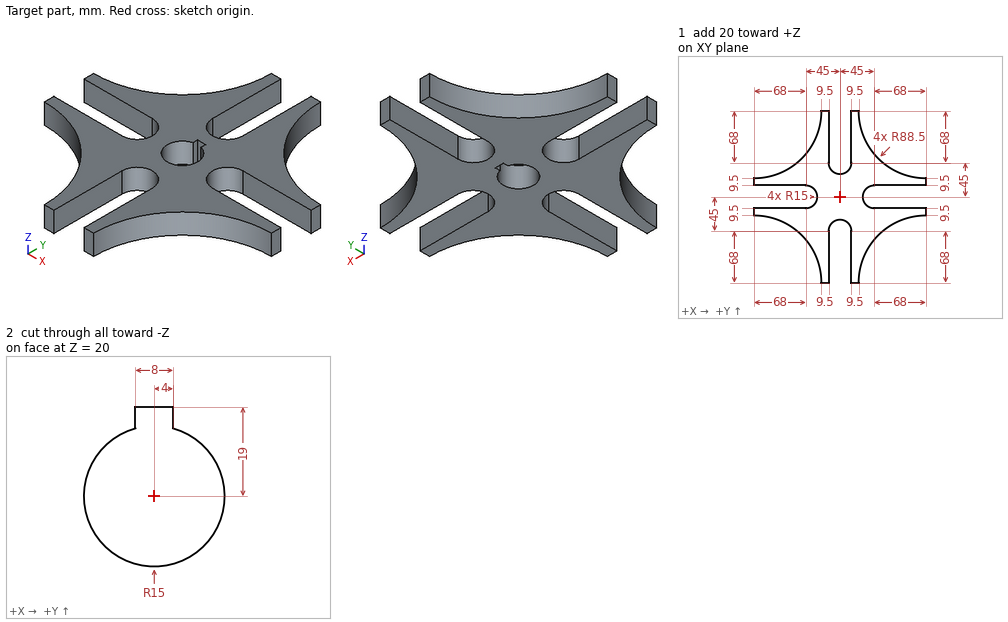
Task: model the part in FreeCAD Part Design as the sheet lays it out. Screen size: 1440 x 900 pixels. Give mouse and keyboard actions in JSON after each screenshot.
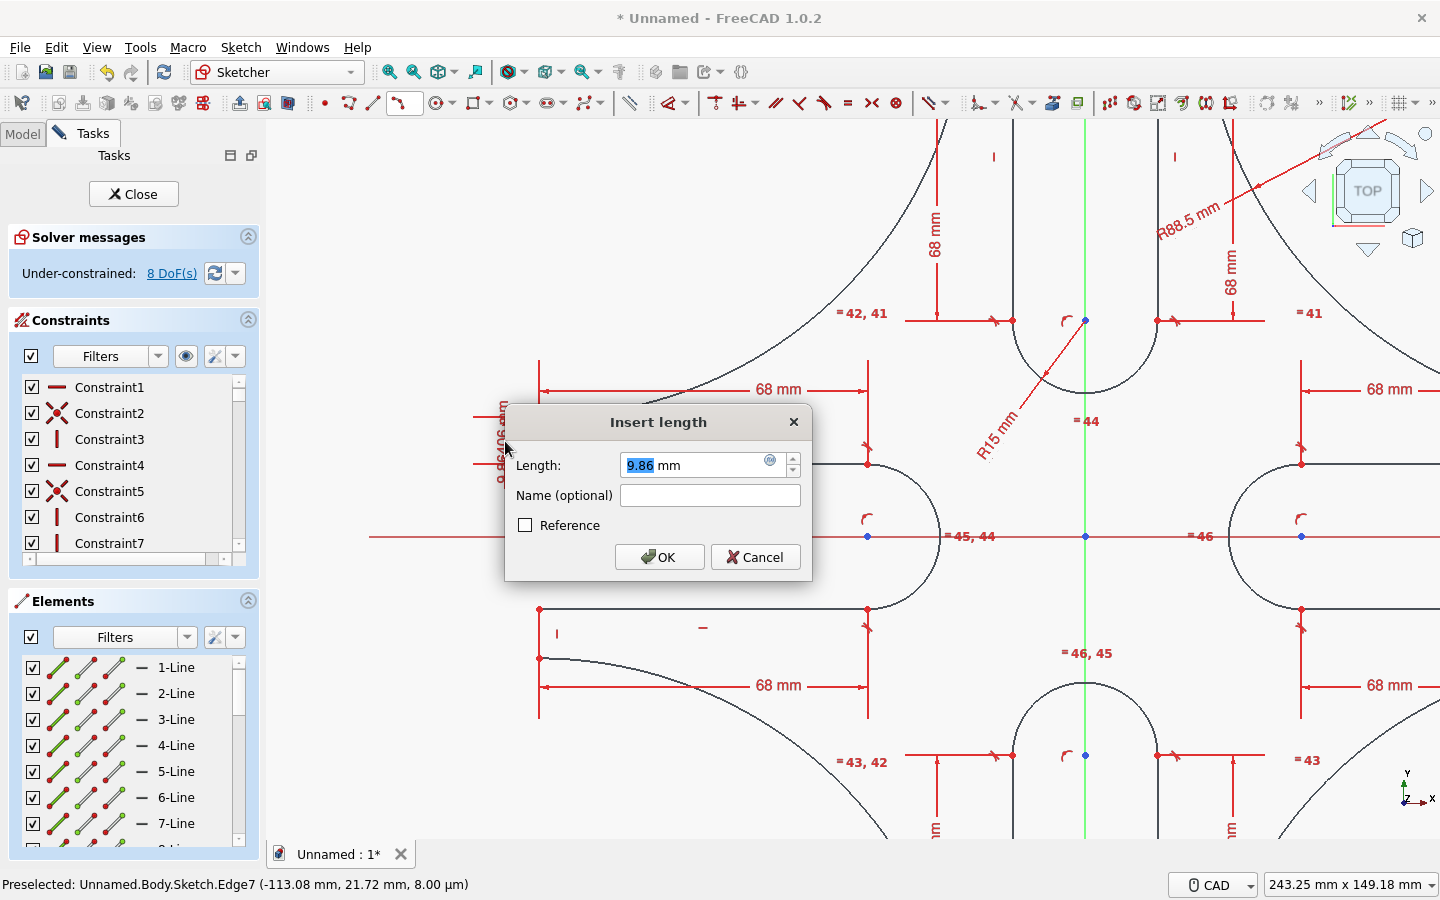
{"action": "type", "text": "9.5"}
{"action": "key", "text": "Return"}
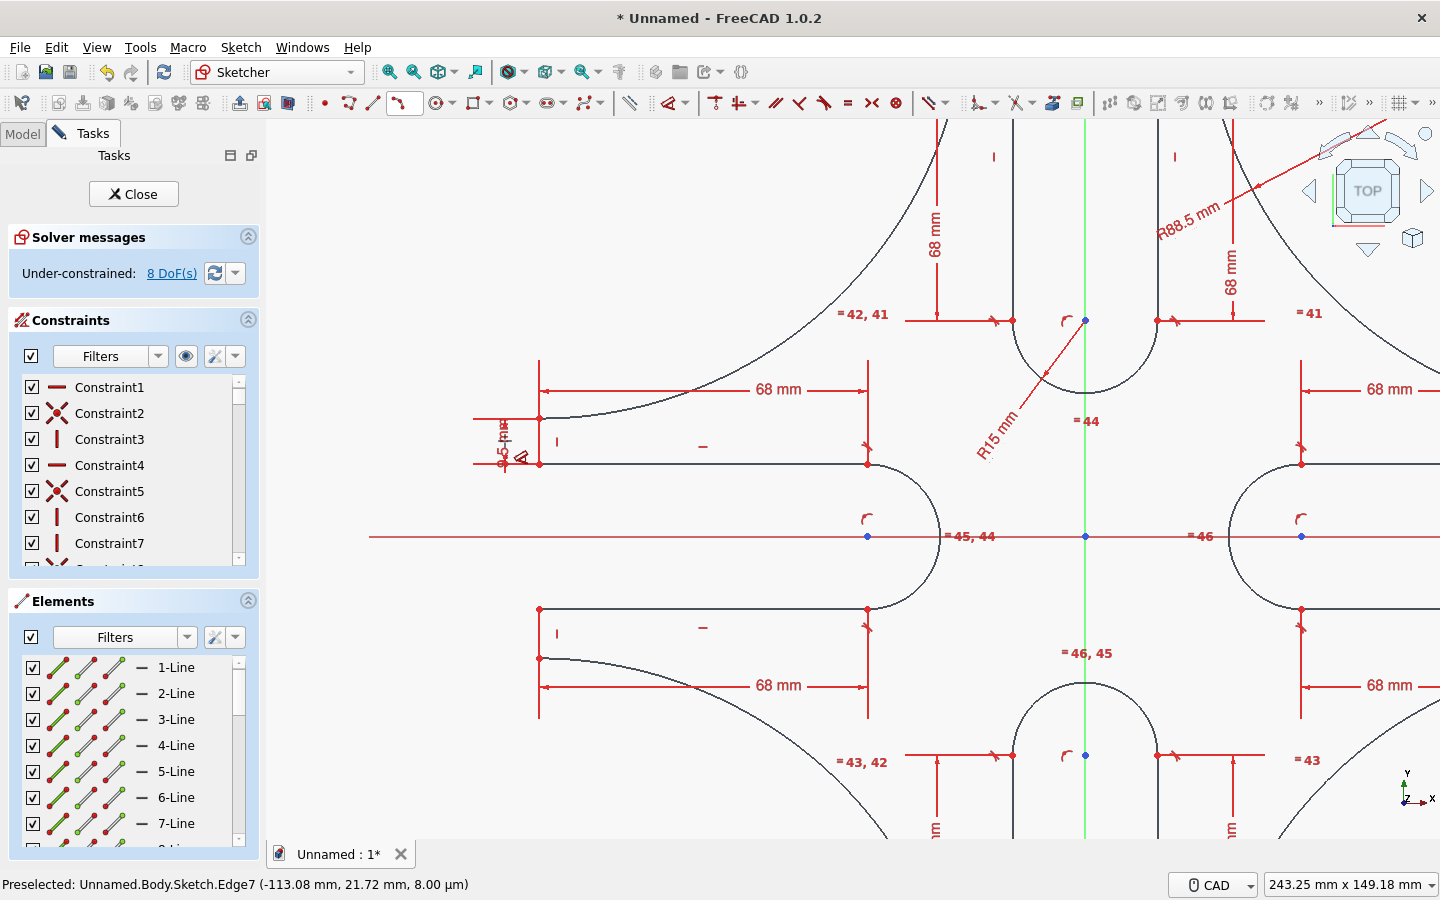
{"action": "left_click", "coordinate": [539, 624]}
{"action": "left_click", "coordinate": [505, 634]}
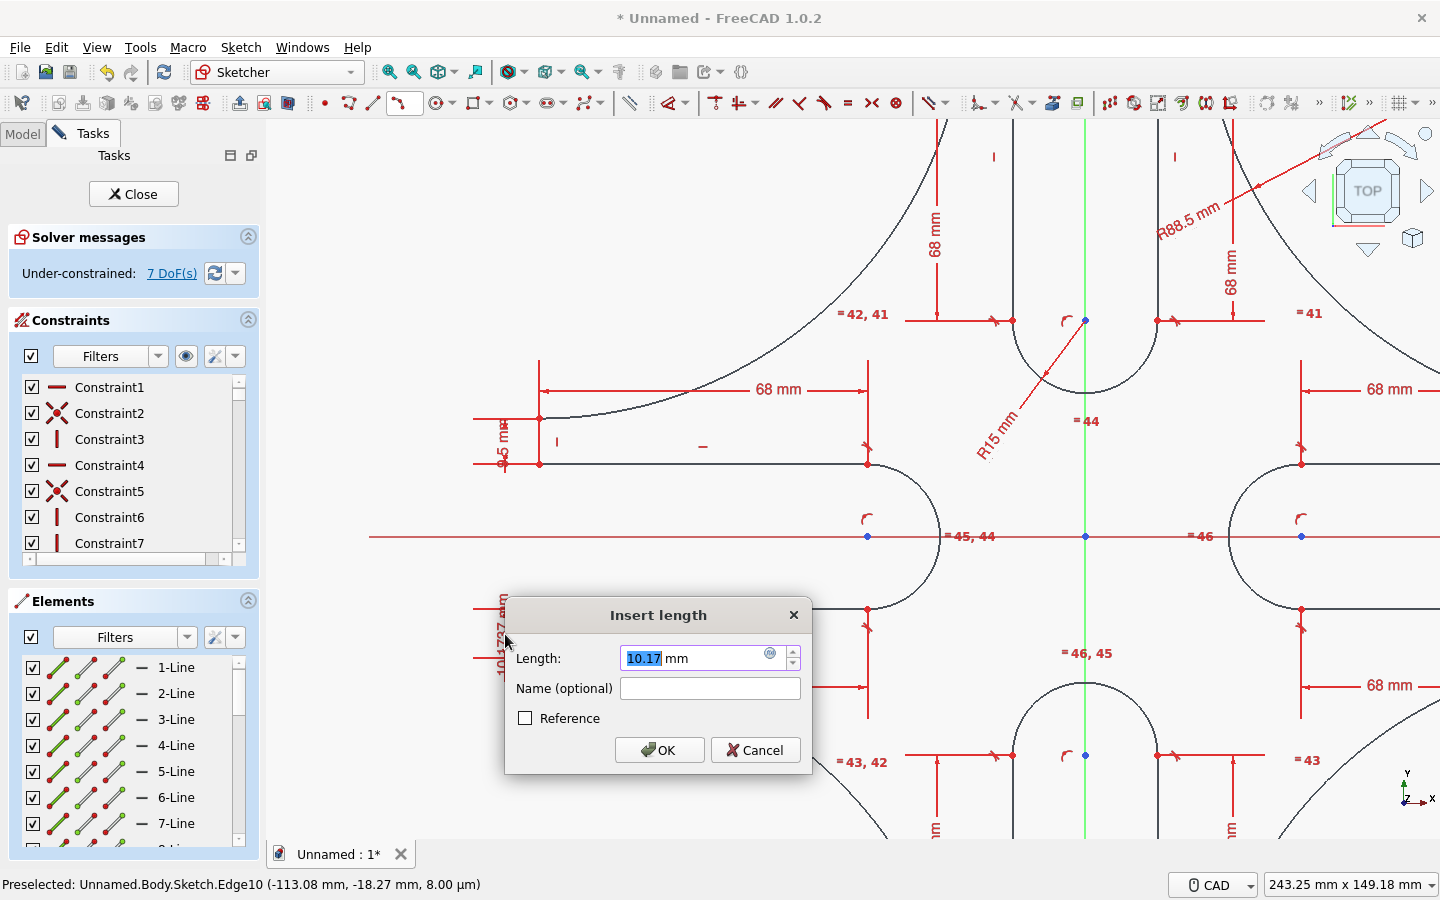
{"action": "type", "text": "9.5"}
{"action": "key", "text": "Return"}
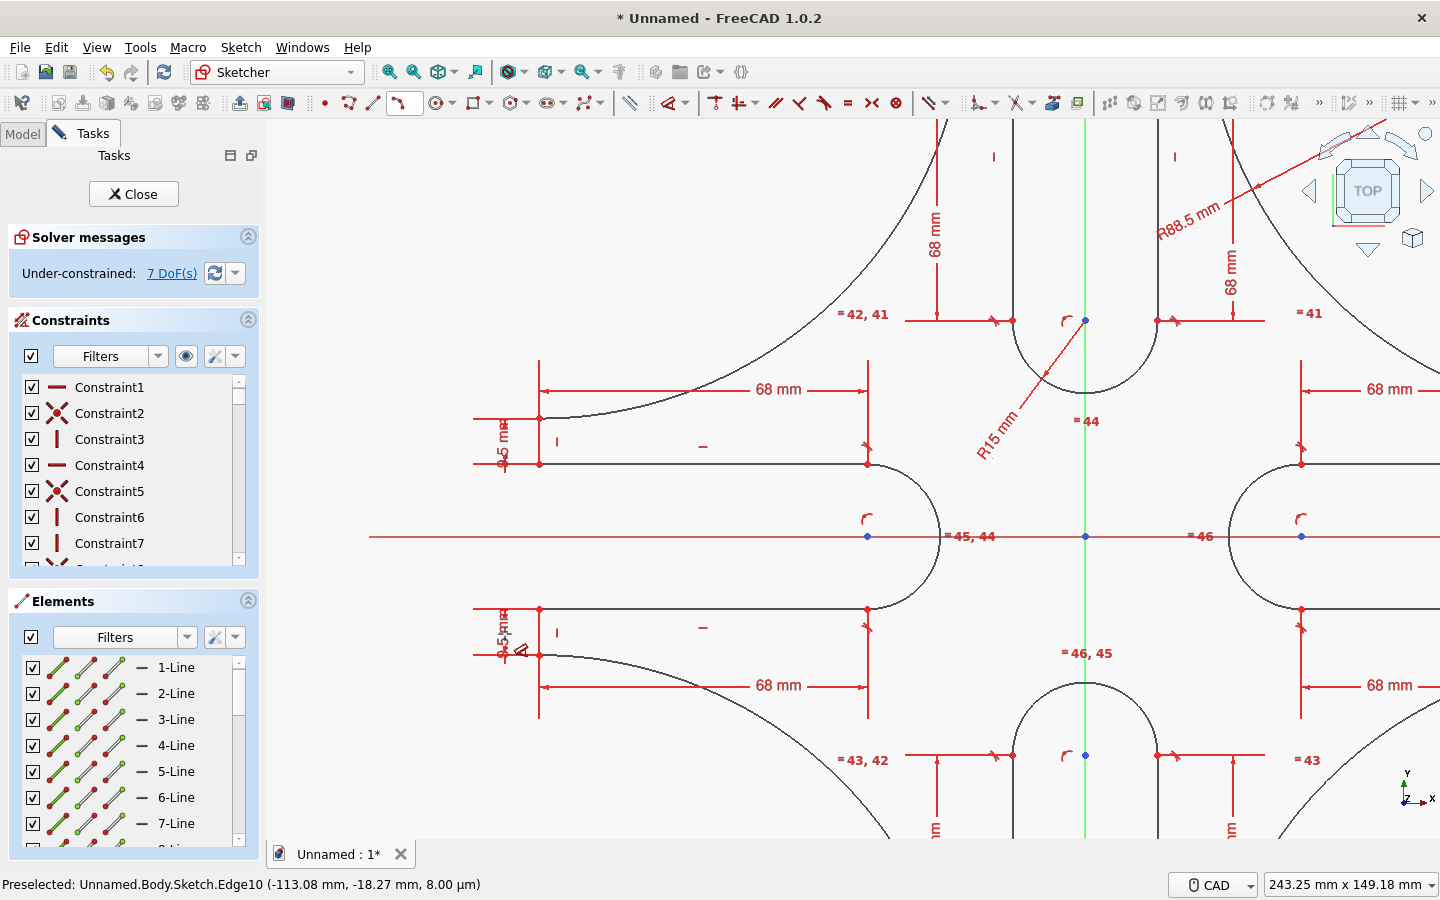
{"action": "scroll", "coordinate": [539, 432], "scroll_direction": "down", "scroll_amount": 4}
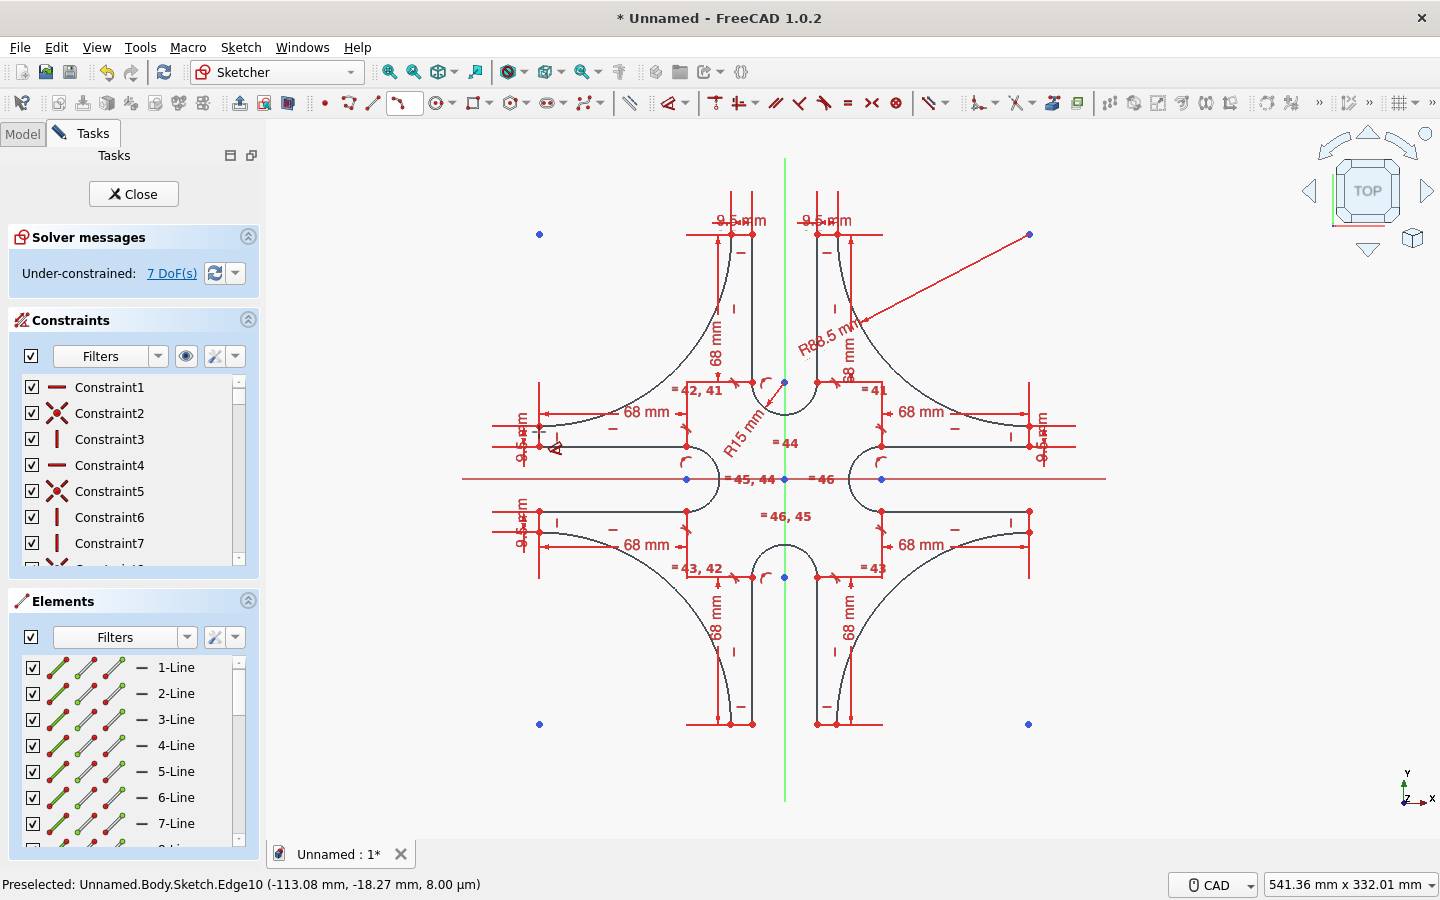
{"action": "scroll", "coordinate": [737, 725], "scroll_direction": "up", "scroll_amount": 4}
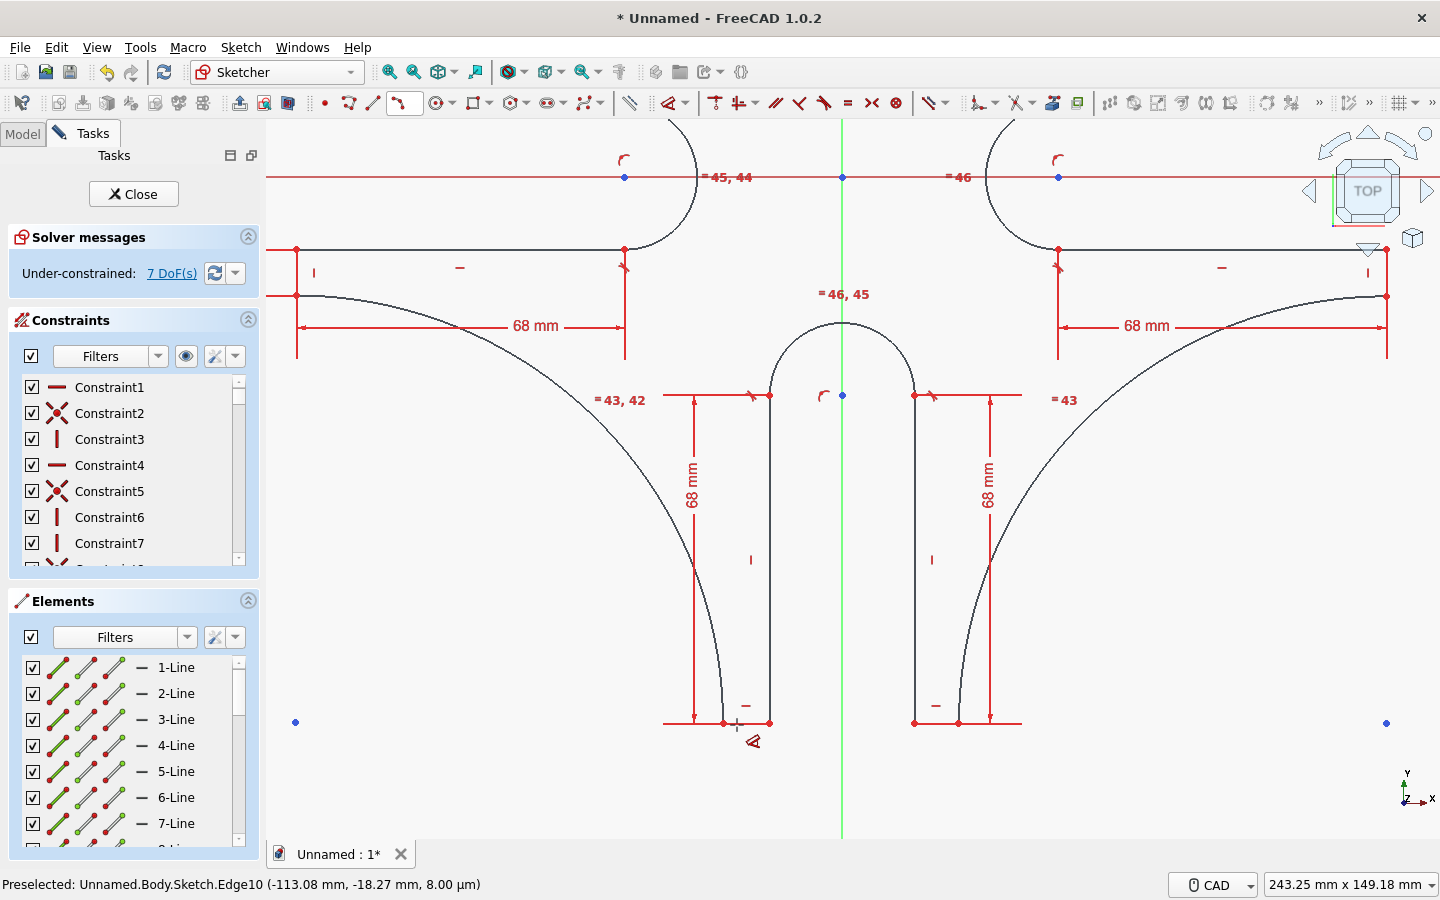
{"action": "left_click", "coordinate": [737, 724]}
{"action": "left_click", "coordinate": [746, 758]}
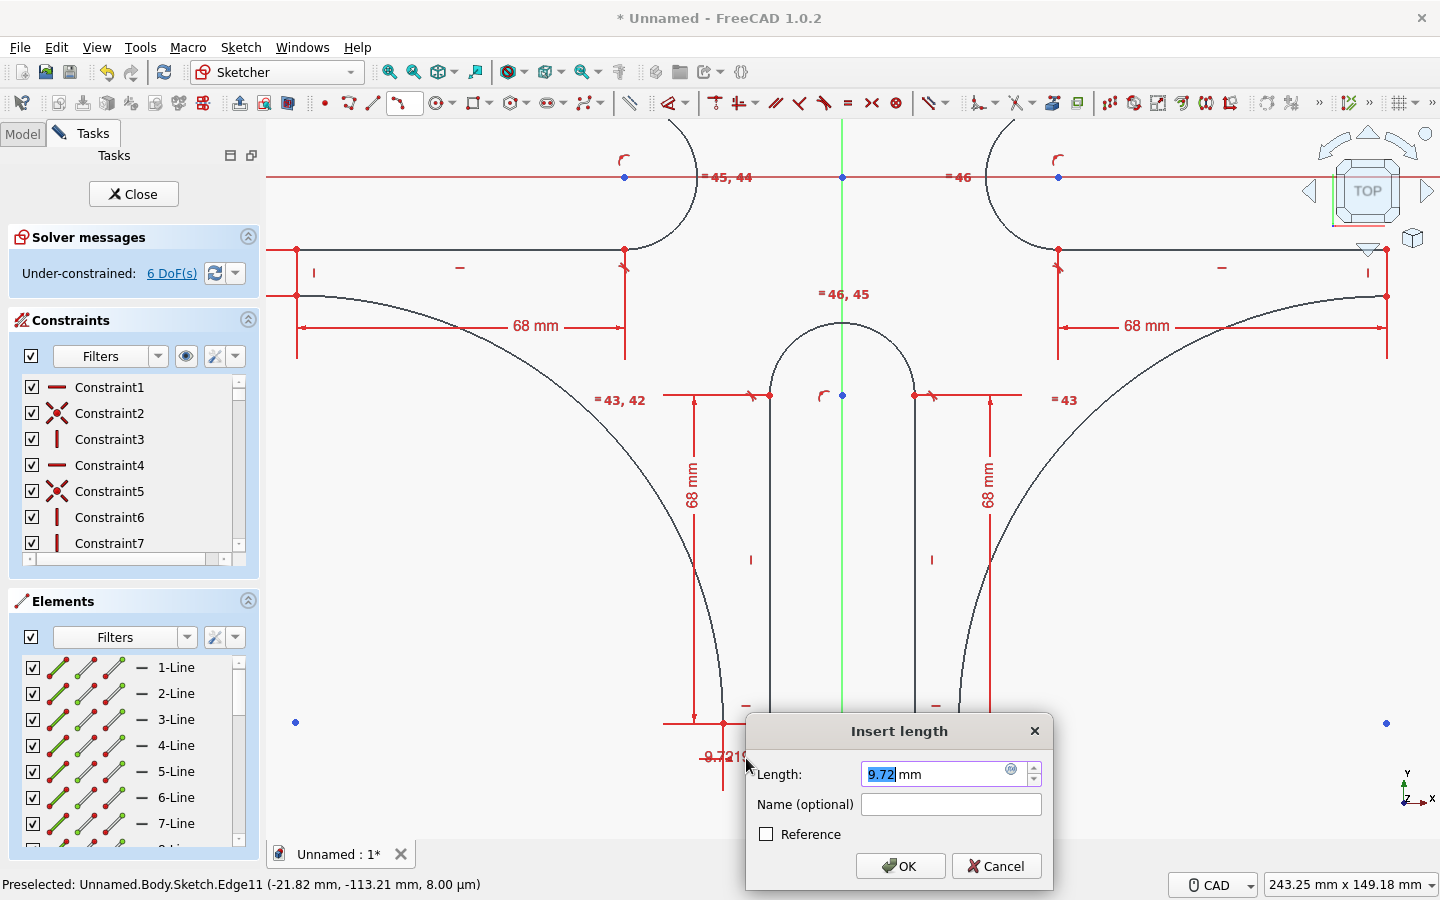
{"action": "type", "text": "9.5"}
{"action": "key", "text": "Return"}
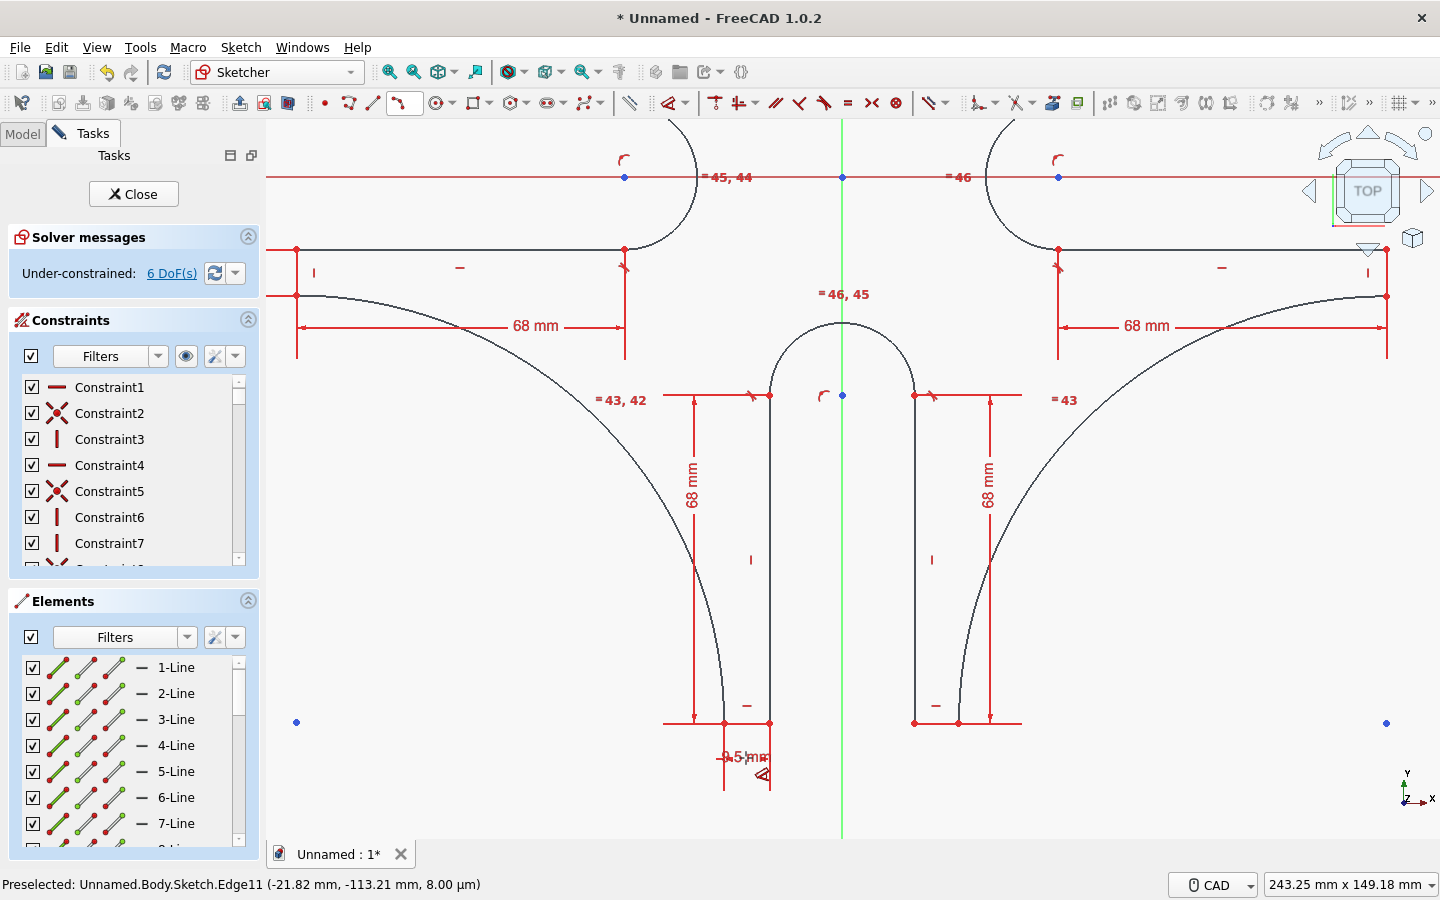
{"action": "left_click", "coordinate": [928, 724]}
{"action": "left_click", "coordinate": [937, 758]}